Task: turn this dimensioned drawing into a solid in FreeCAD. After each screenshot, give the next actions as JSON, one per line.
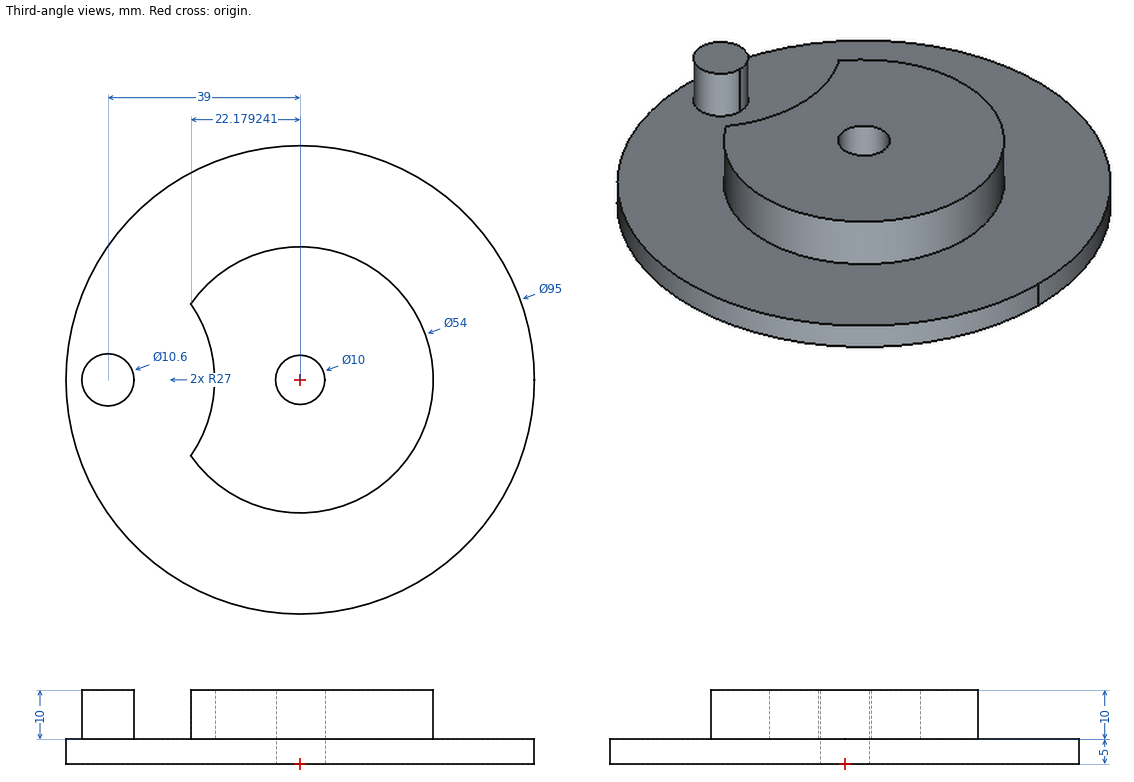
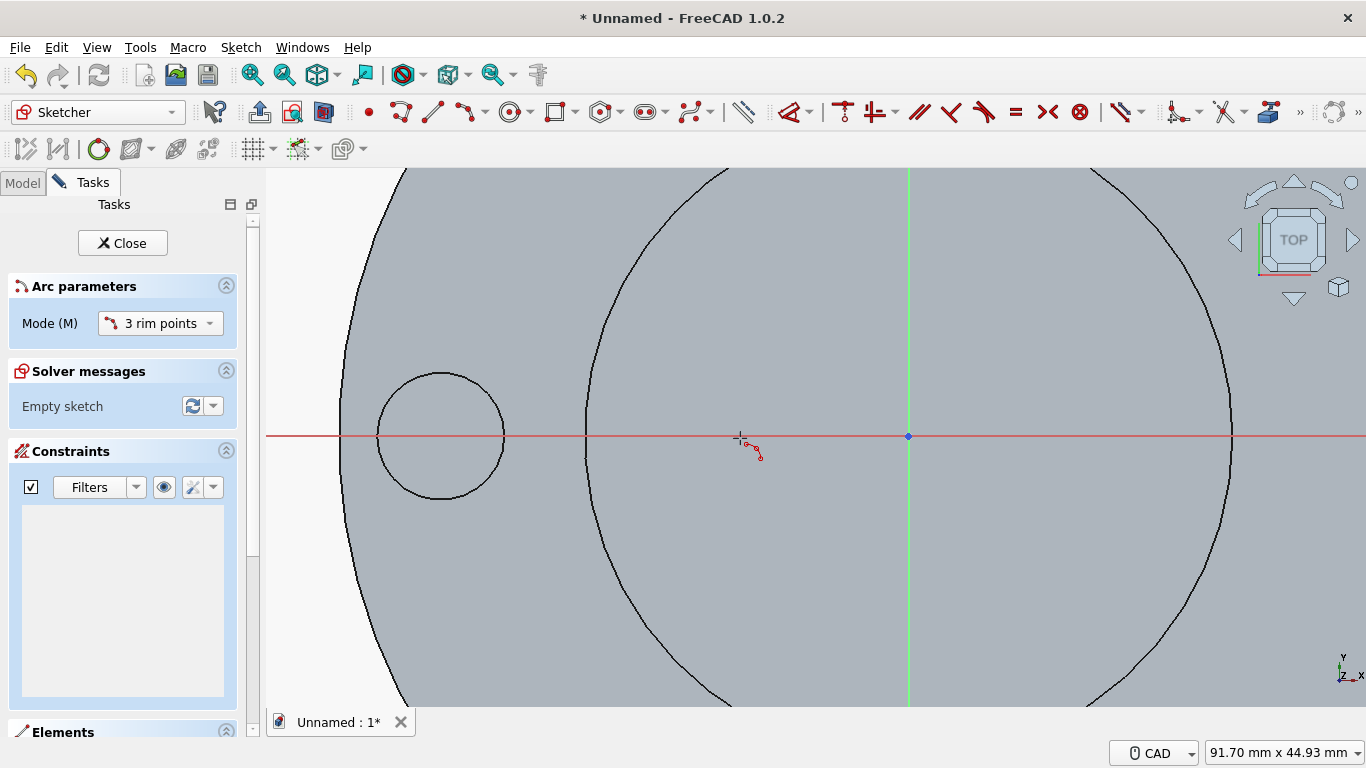
{"action": "left_click", "coordinate": [643, 252]}
{"action": "left_click", "coordinate": [643, 621]}
{"action": "left_click", "coordinate": [587, 397]}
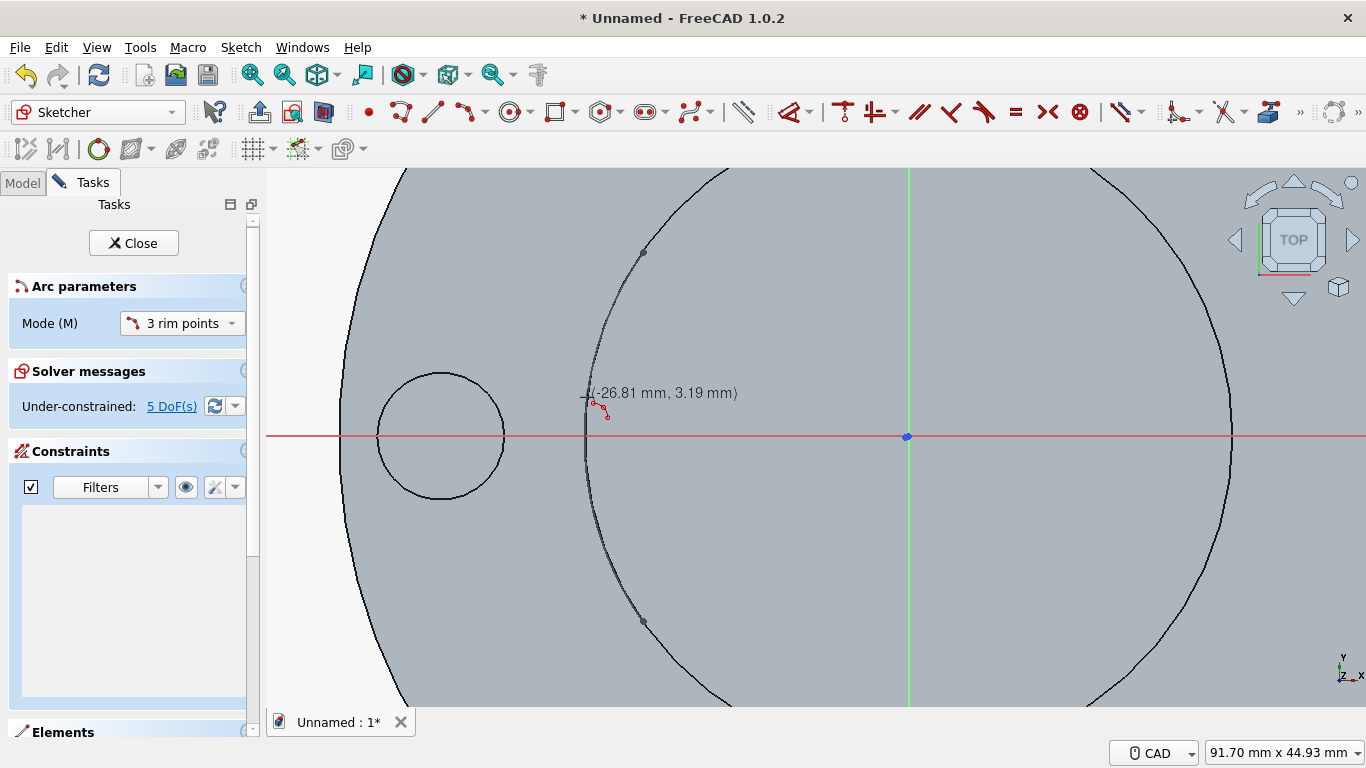
{"action": "left_click", "coordinate": [643, 622]}
{"action": "left_click", "coordinate": [643, 253]}
{"action": "left_click", "coordinate": [698, 475]}
{"action": "key", "text": "Escape"}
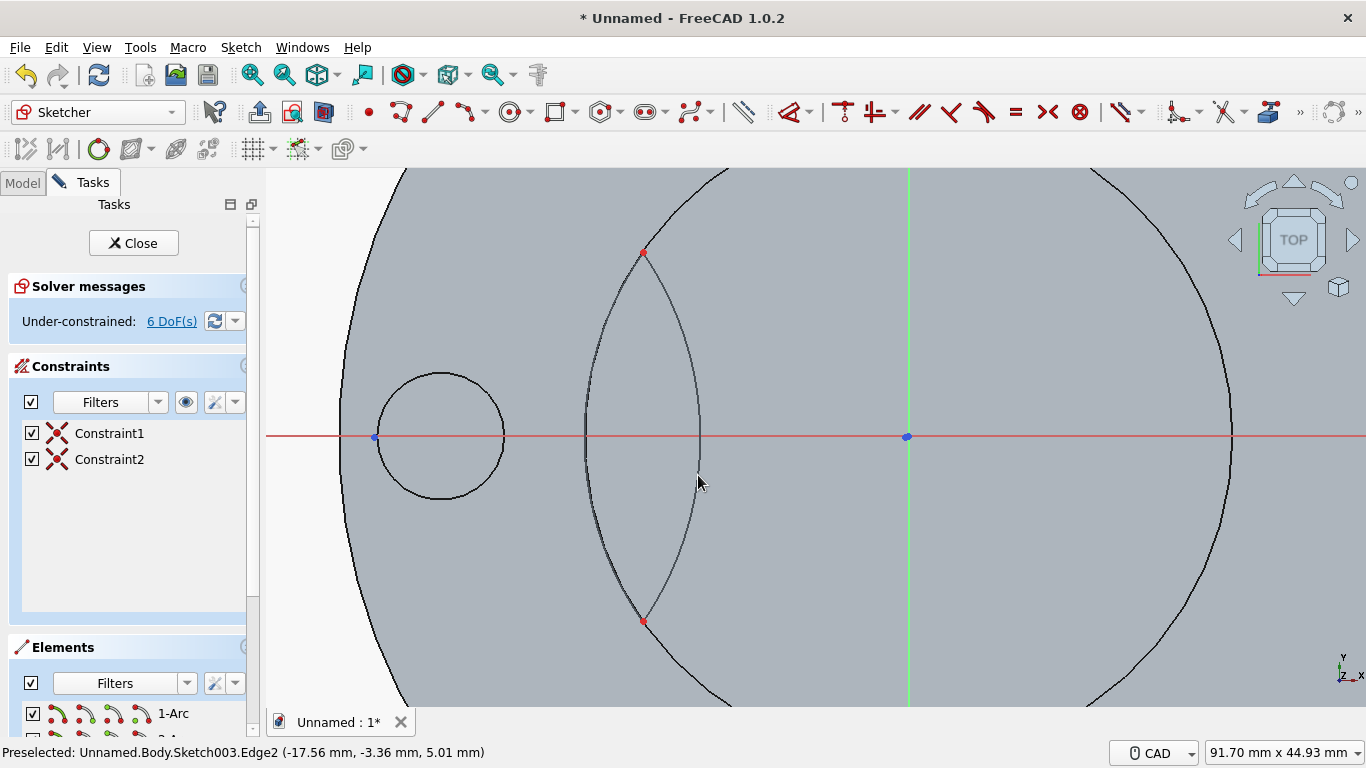
{"action": "left_click_drag", "start_coordinate": [895, 426], "coordinate": [919, 448]}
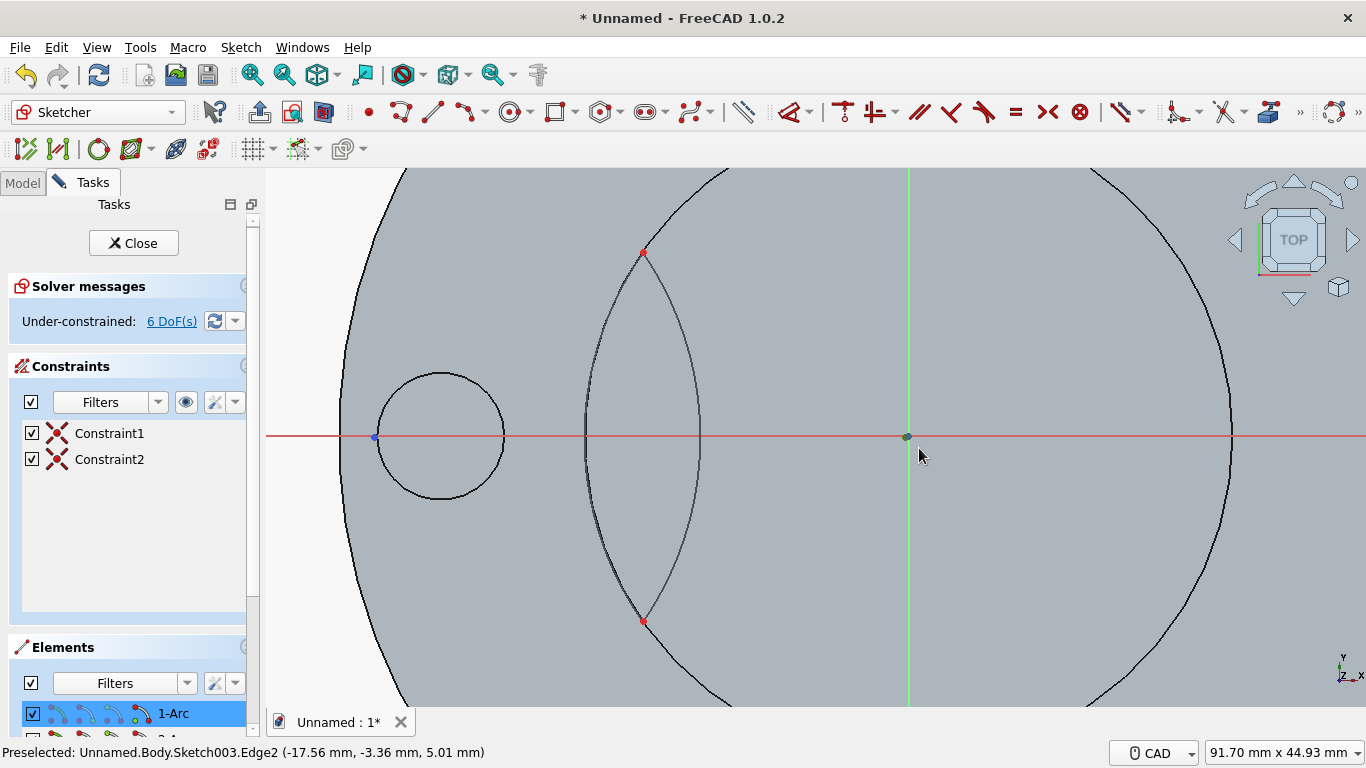
{"action": "left_click", "coordinate": [844, 112]}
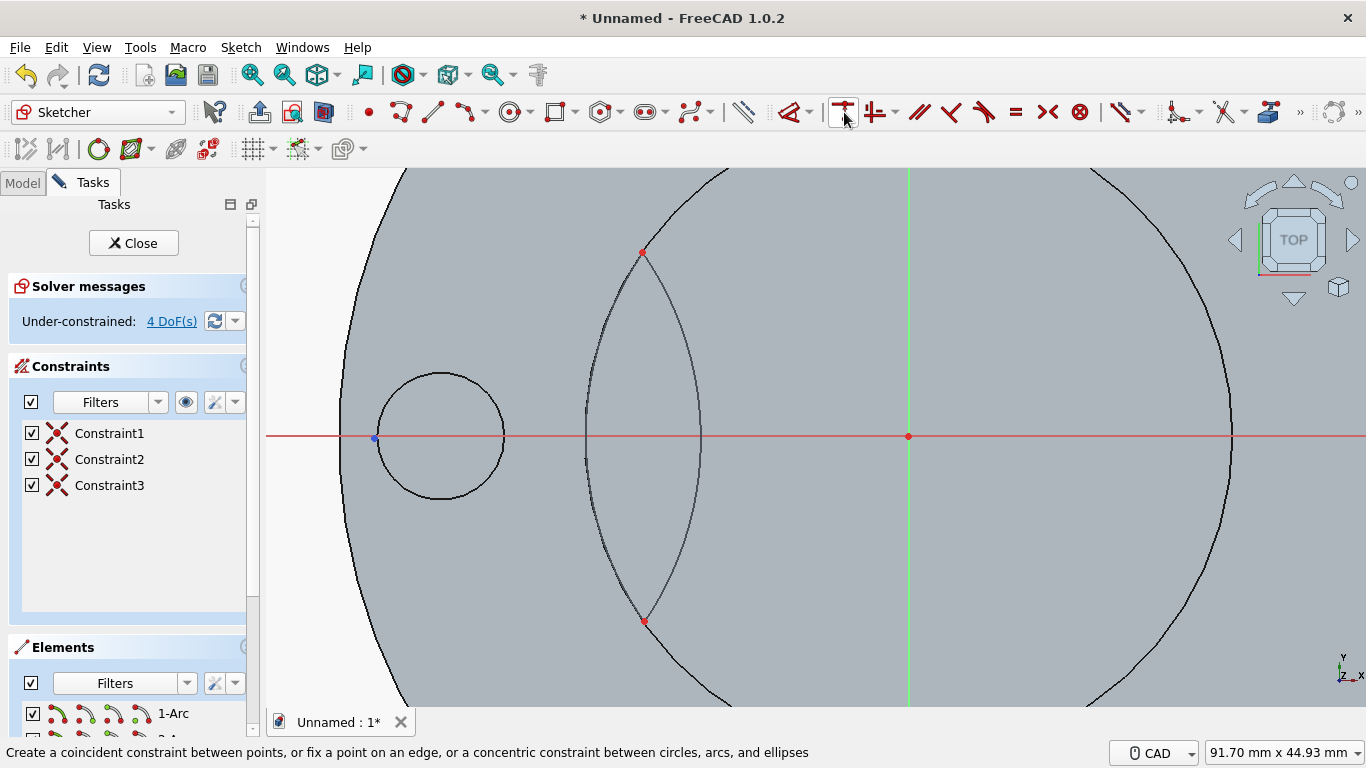
{"action": "left_click", "coordinate": [595, 360]}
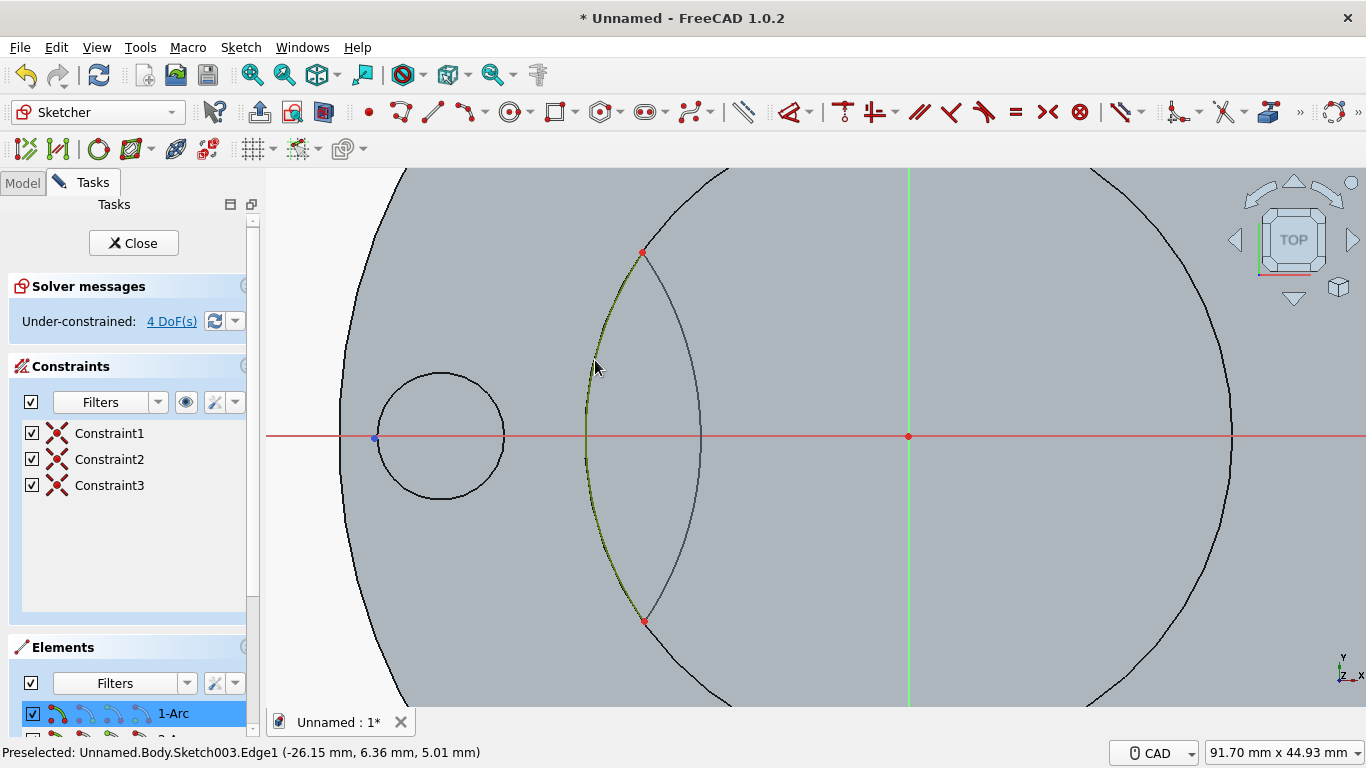
{"action": "left_click", "coordinate": [692, 515]}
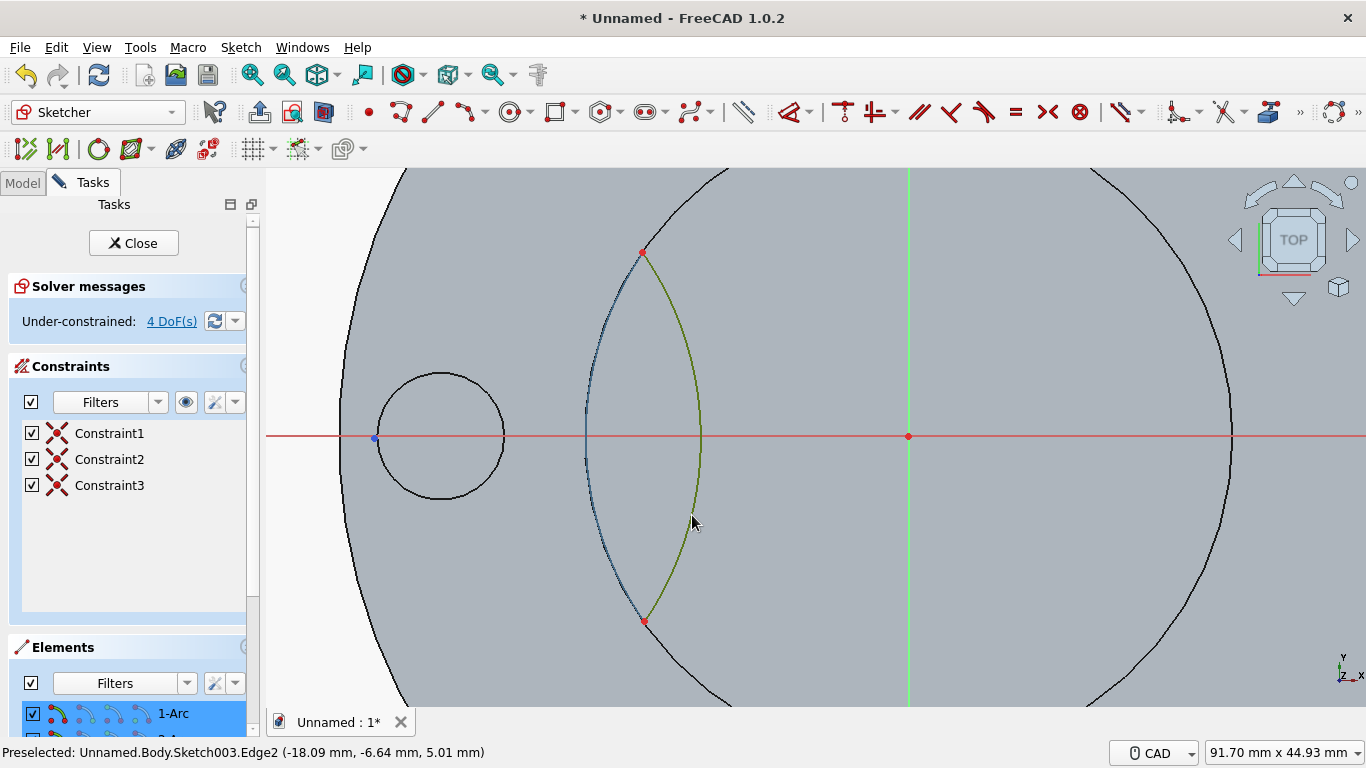
{"action": "key", "text": "e"}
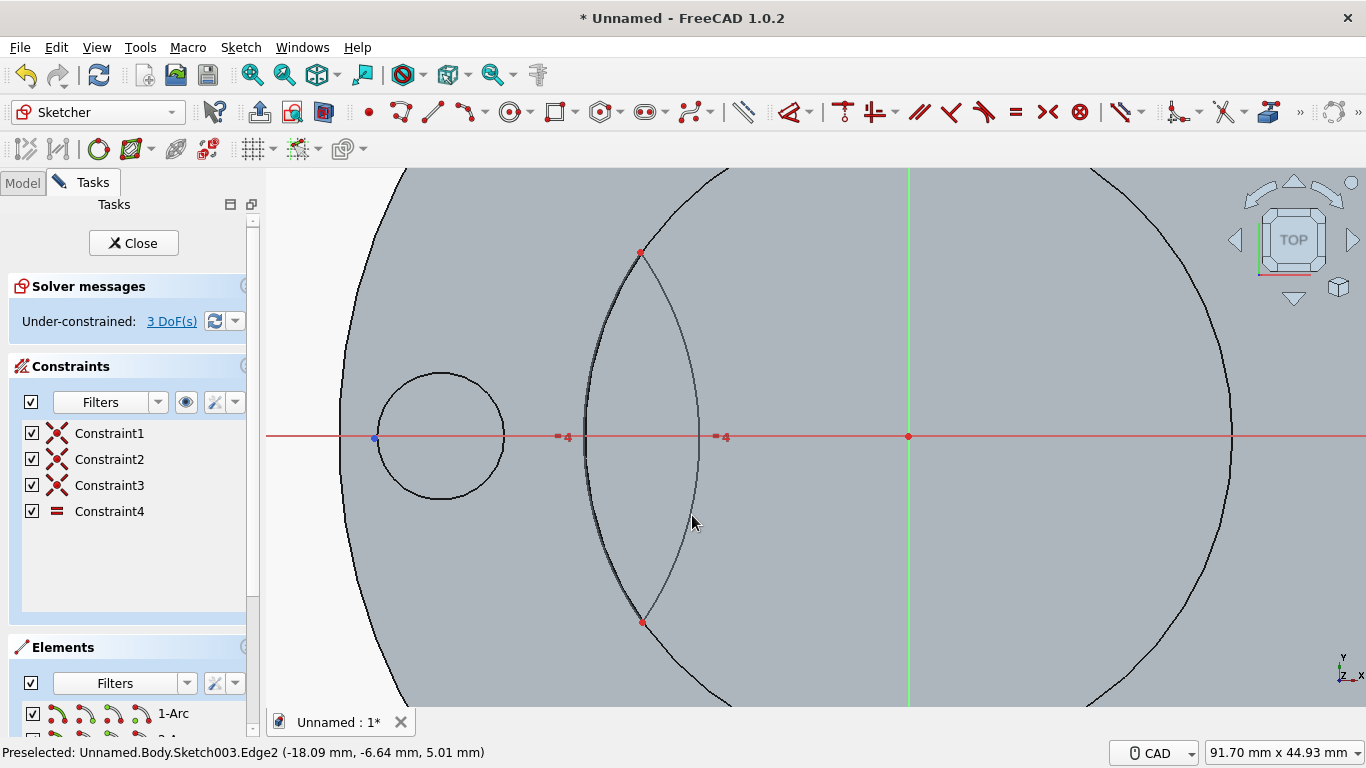
{"action": "left_click", "coordinate": [375, 439]}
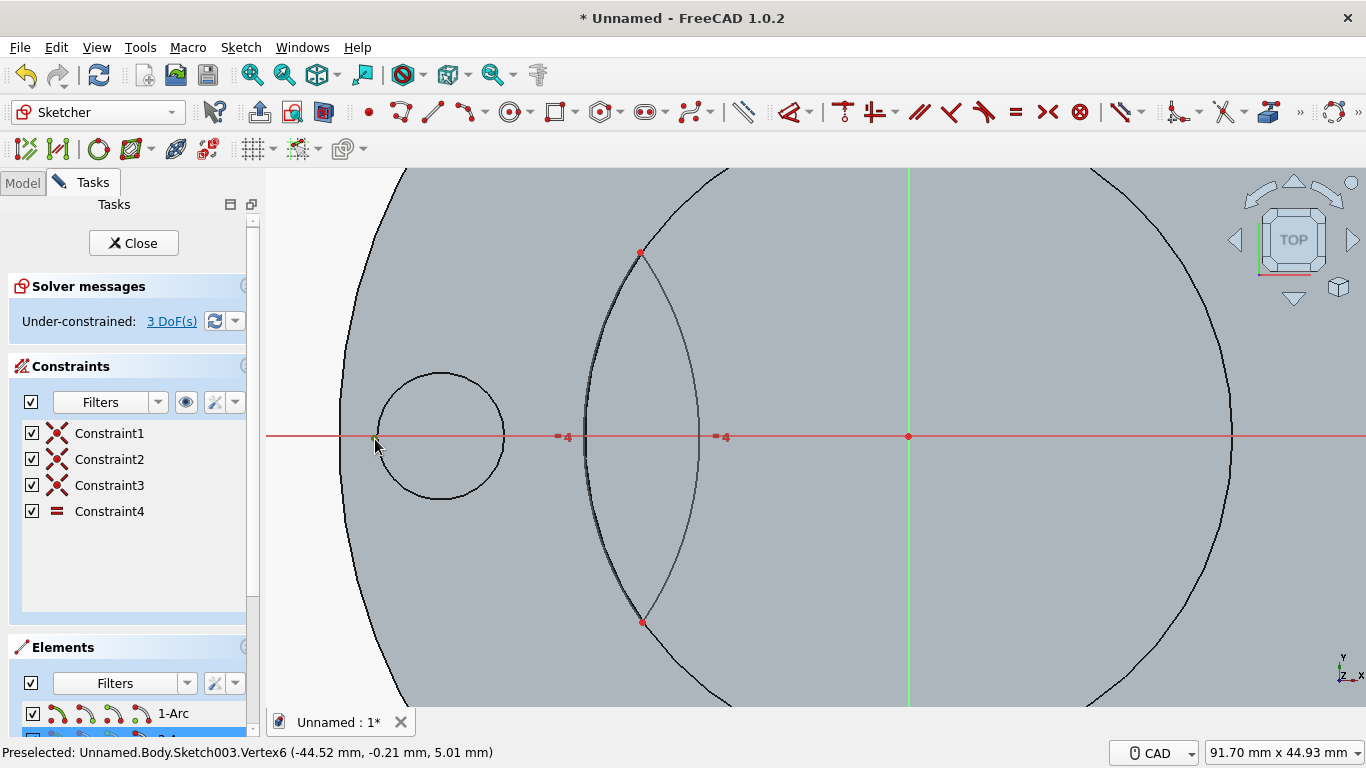
{"action": "left_click", "coordinate": [359, 436]}